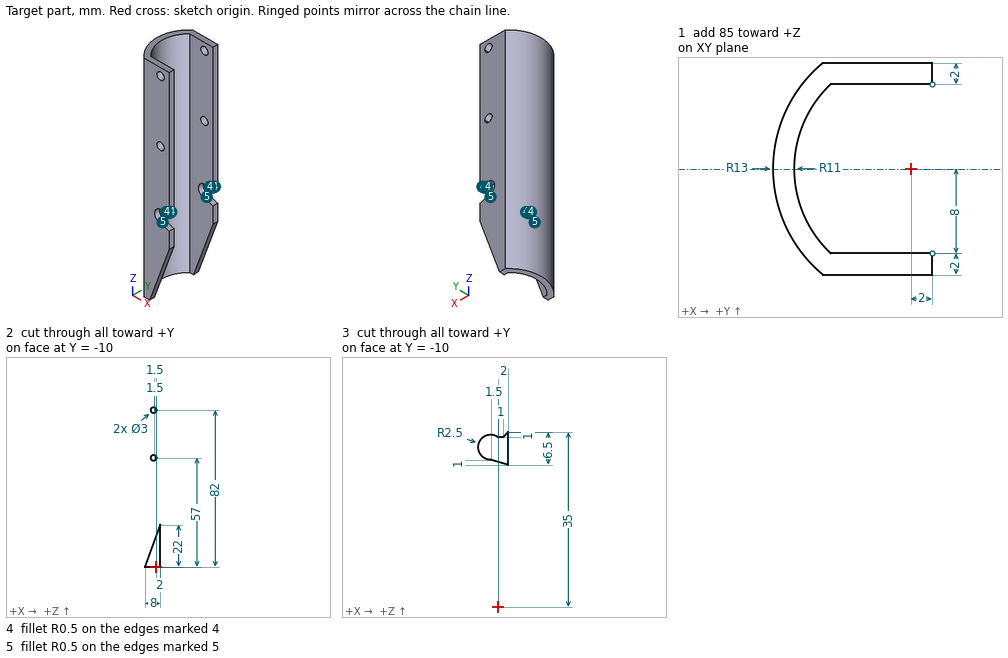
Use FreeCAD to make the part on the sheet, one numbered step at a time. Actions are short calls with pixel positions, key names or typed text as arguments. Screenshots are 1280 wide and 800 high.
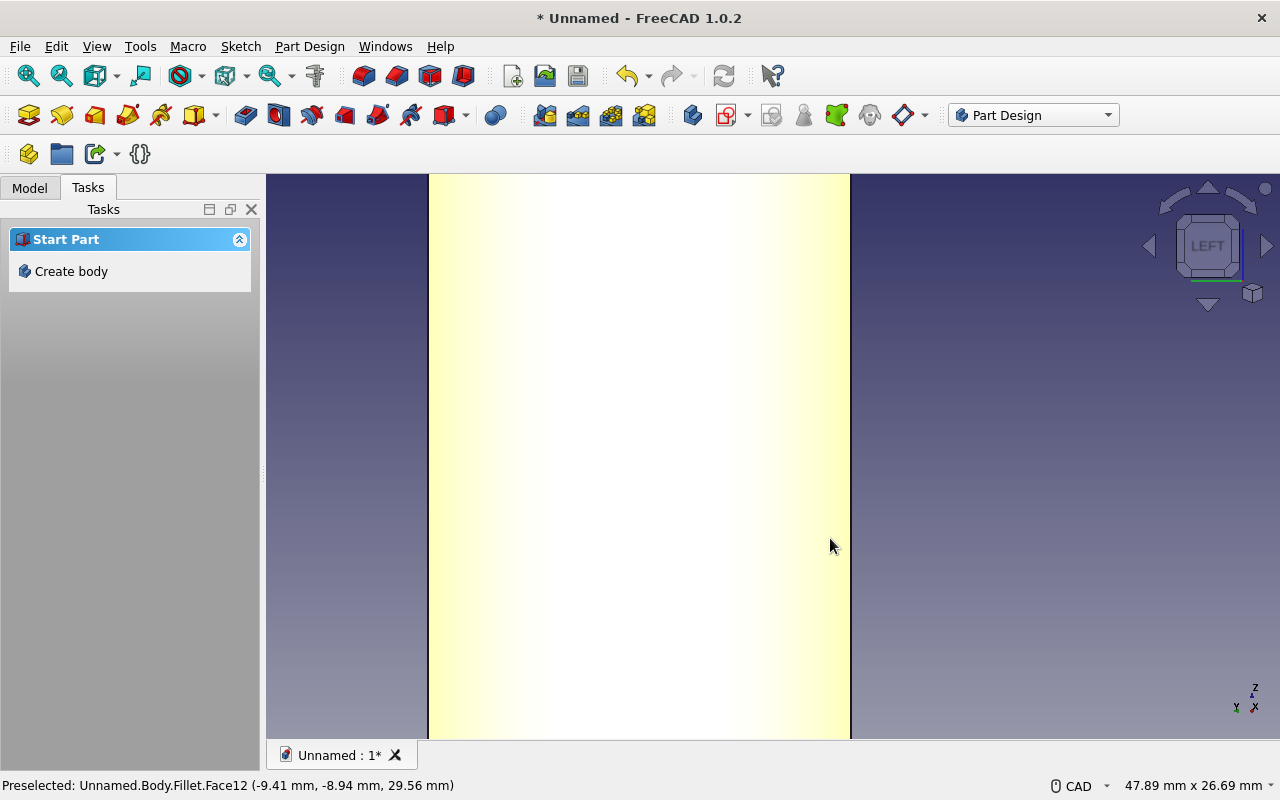
click(29, 76)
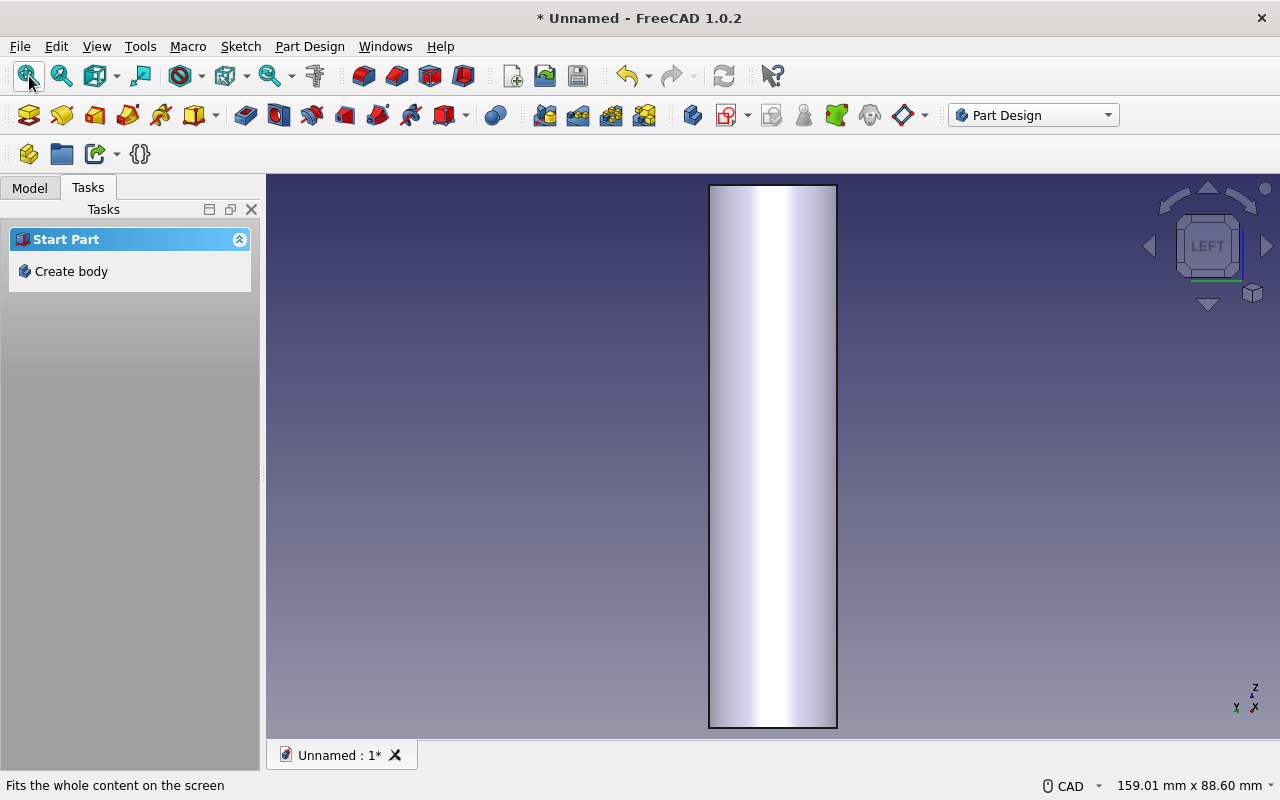
key(v)
key(3)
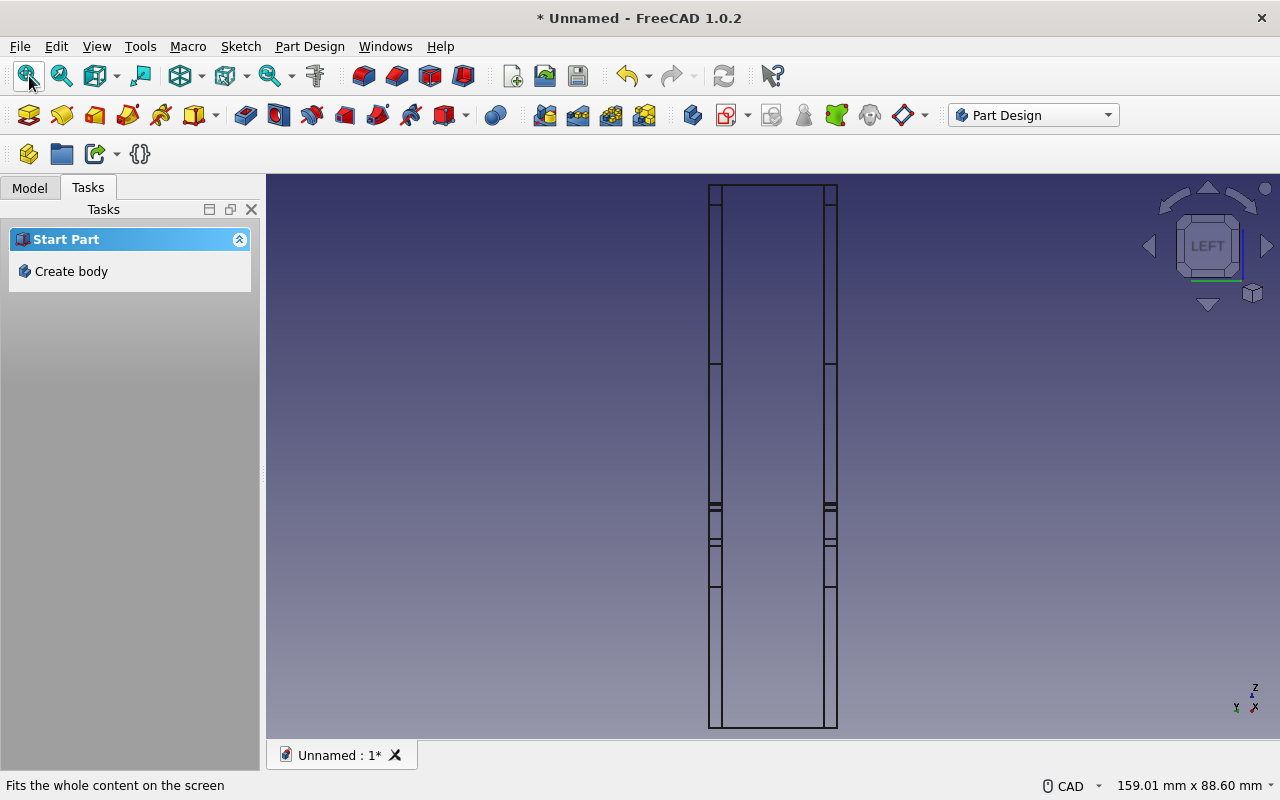
key(0)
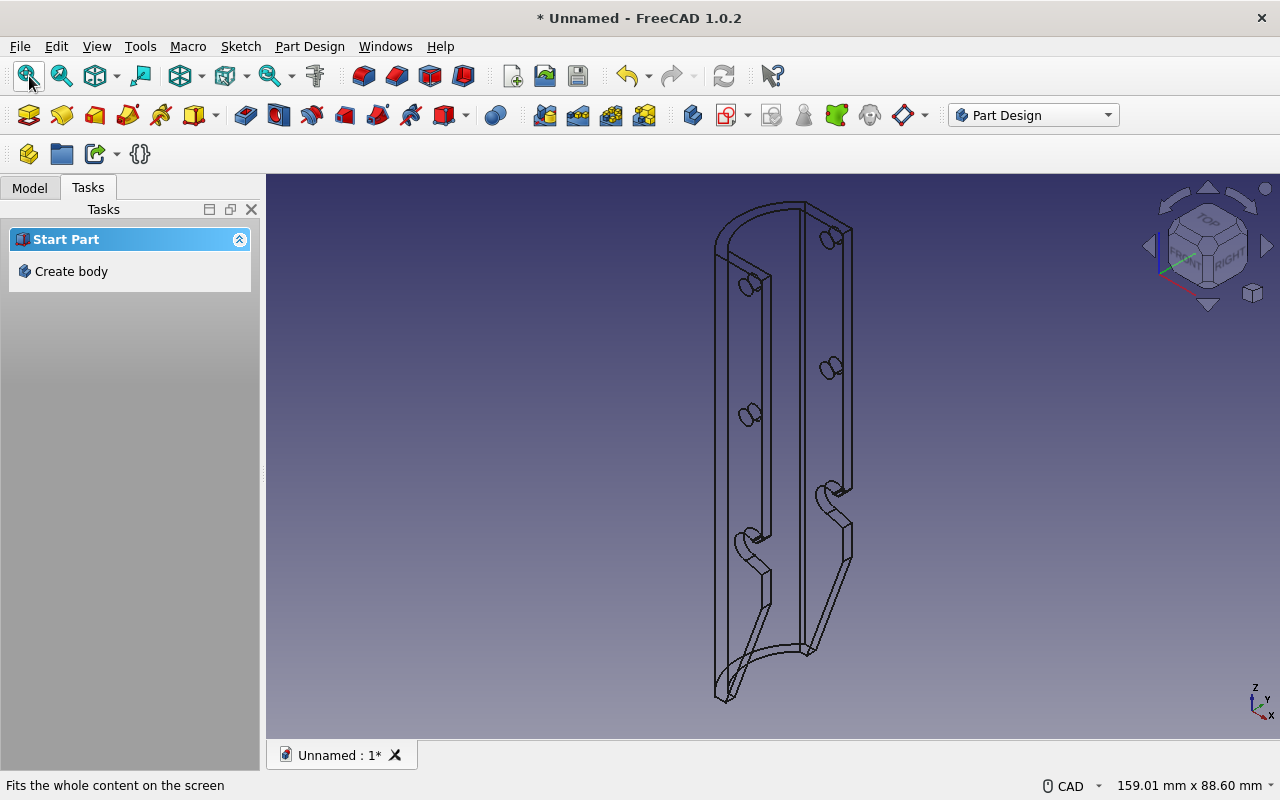
click(752, 556)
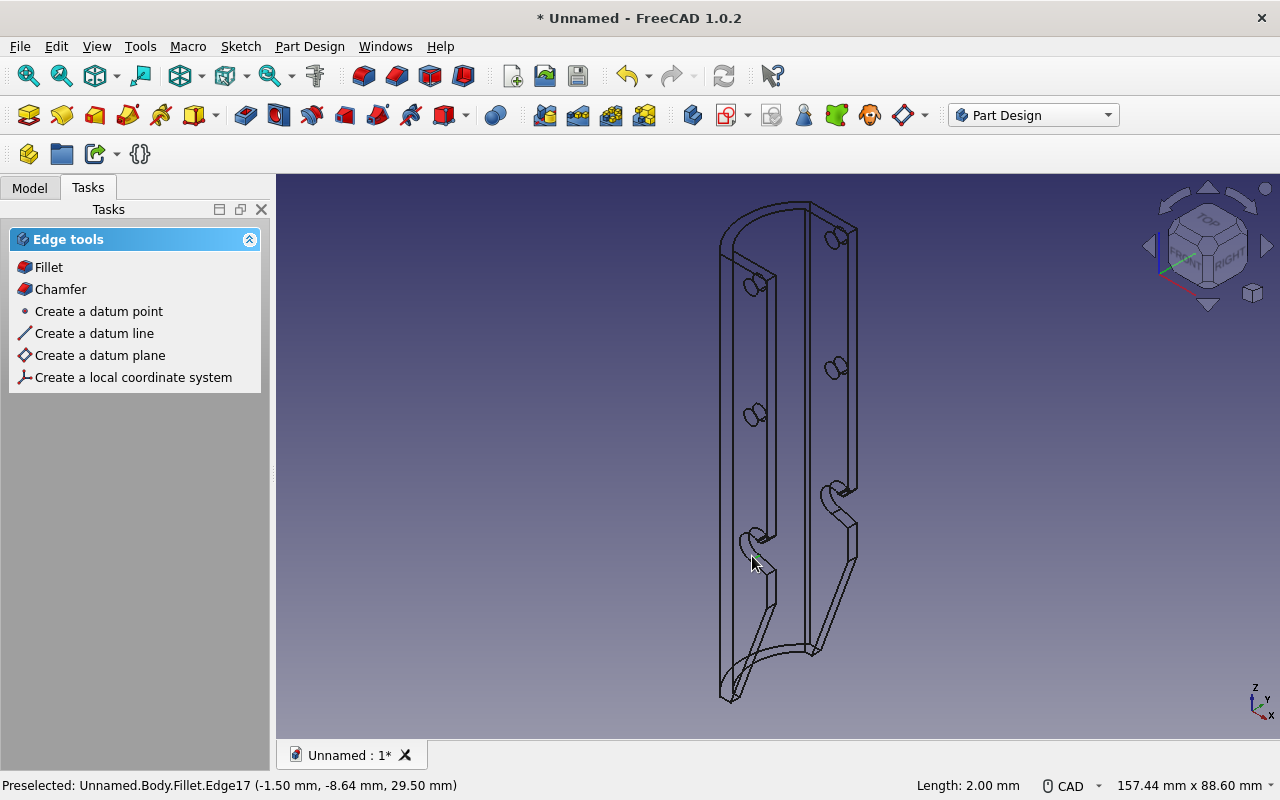
click(838, 509, ctrl)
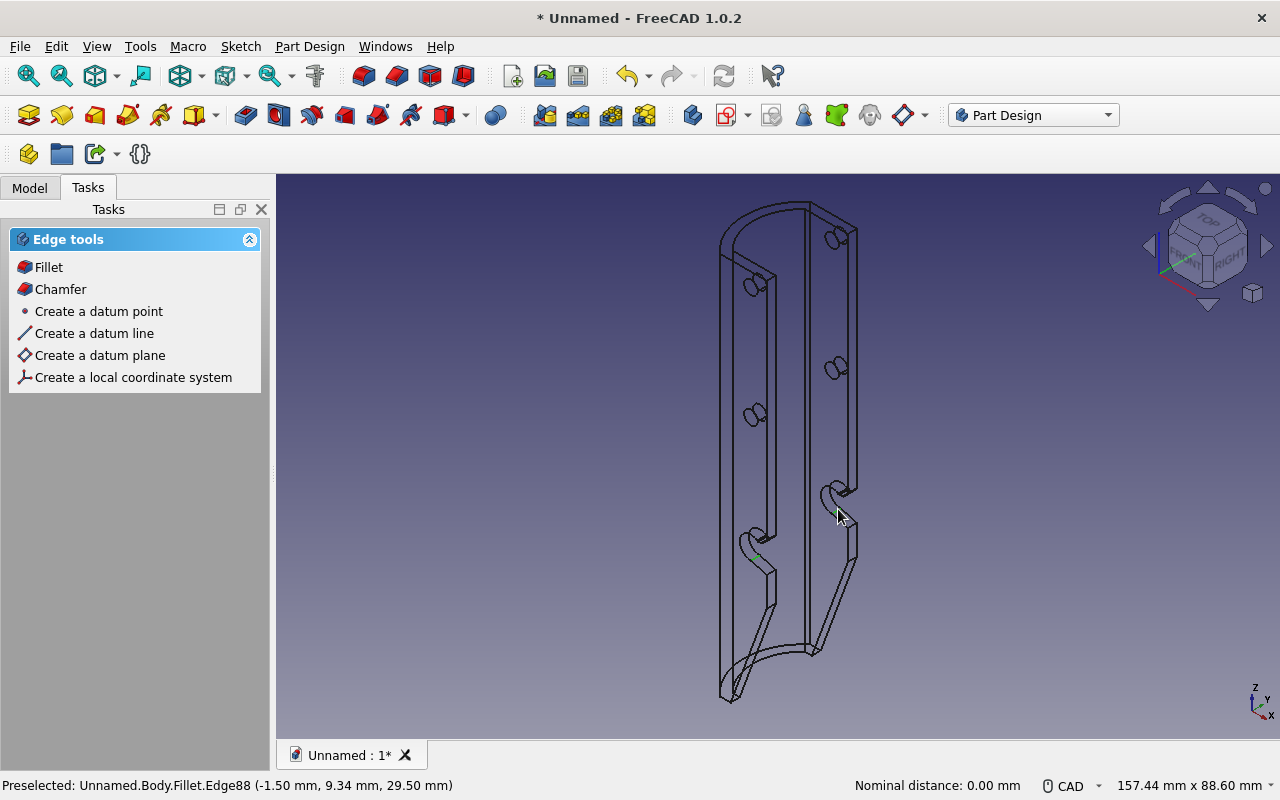
key(v)
key(1)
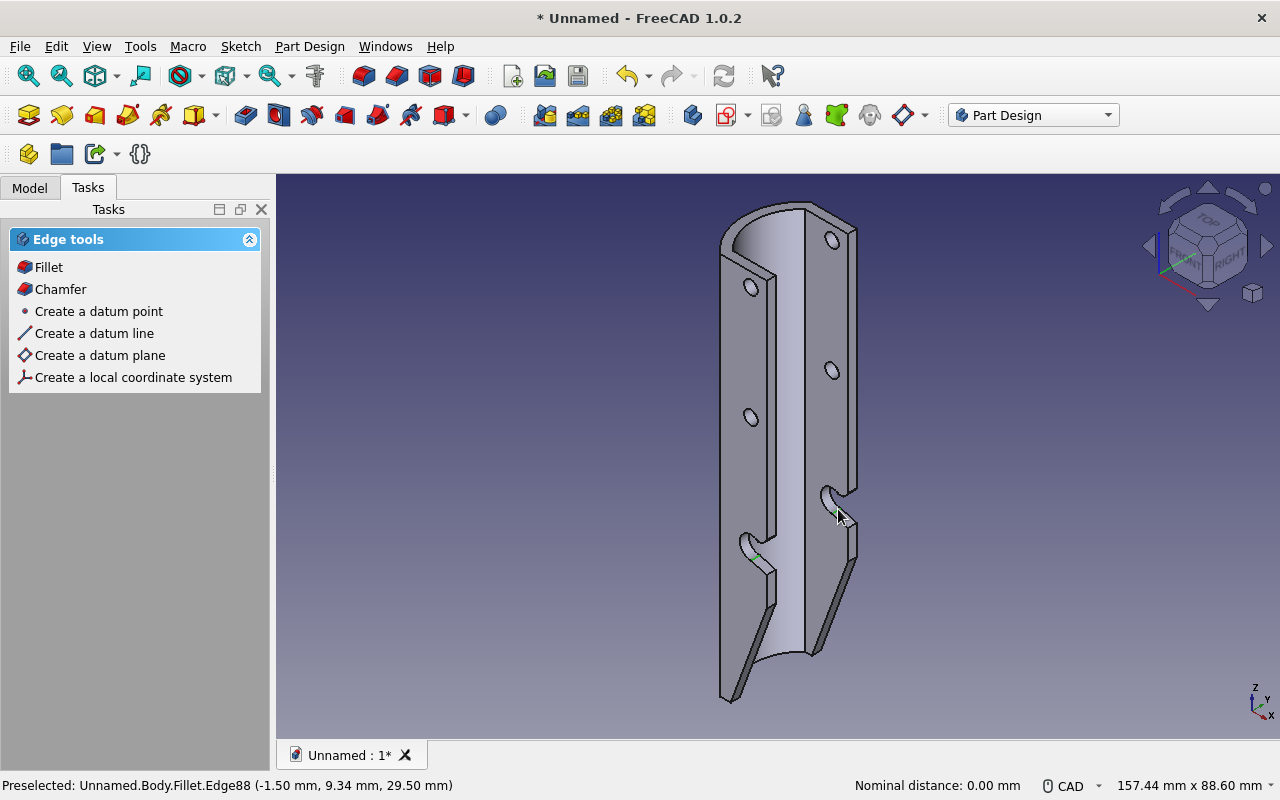
click(364, 76)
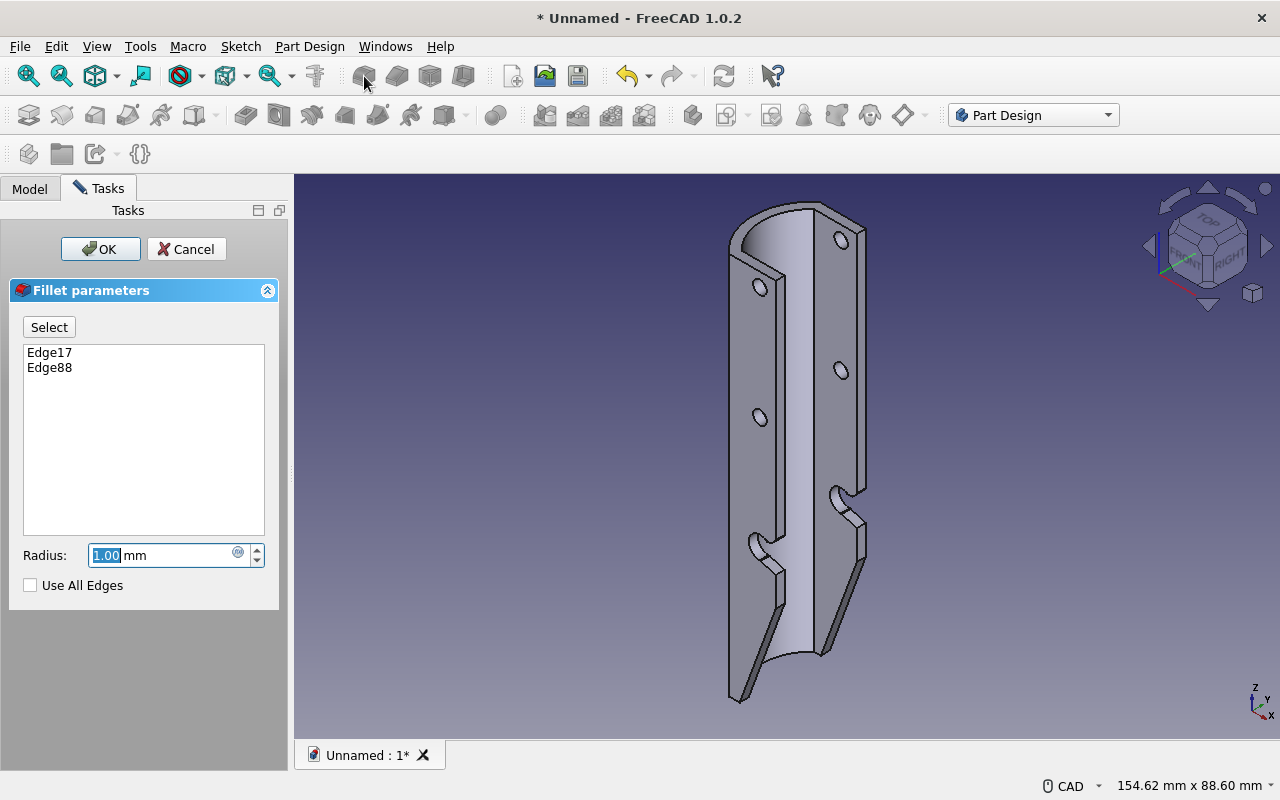
text(0.5)
key(Tab)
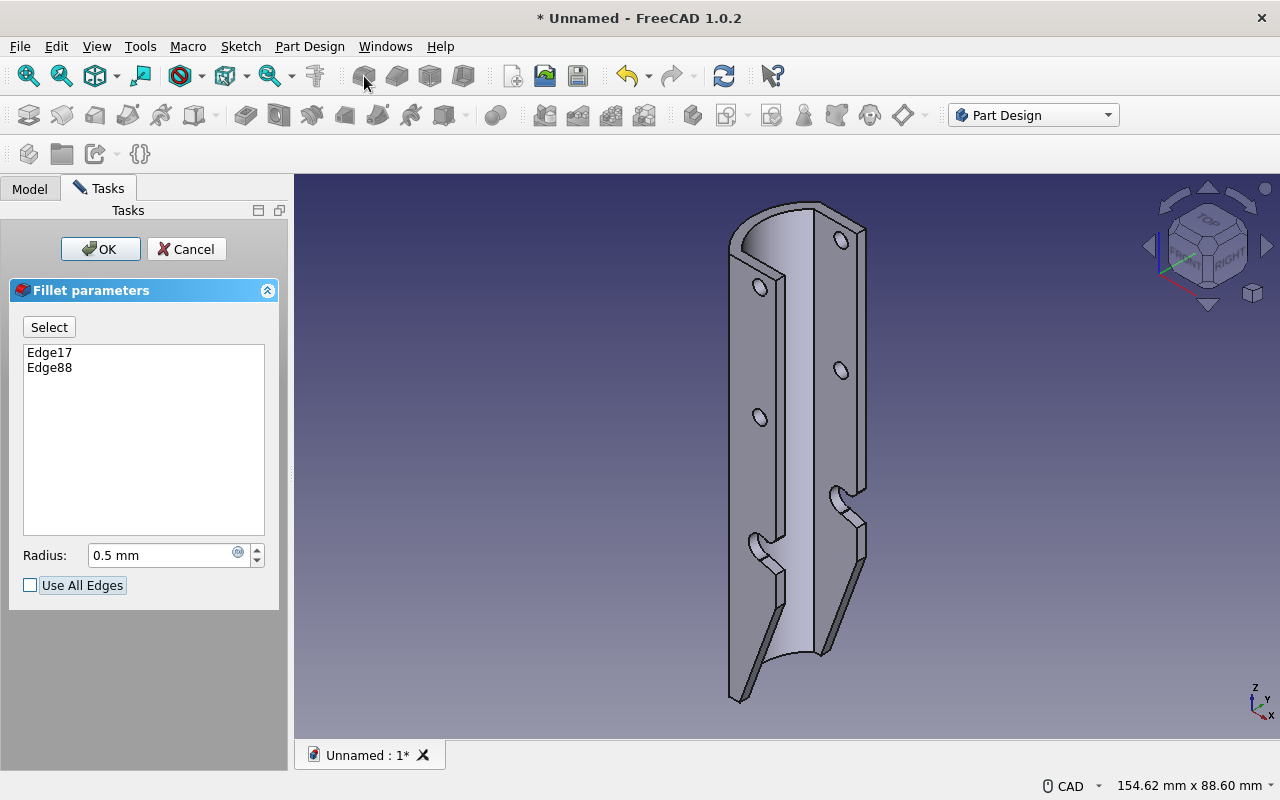
click(101, 249)